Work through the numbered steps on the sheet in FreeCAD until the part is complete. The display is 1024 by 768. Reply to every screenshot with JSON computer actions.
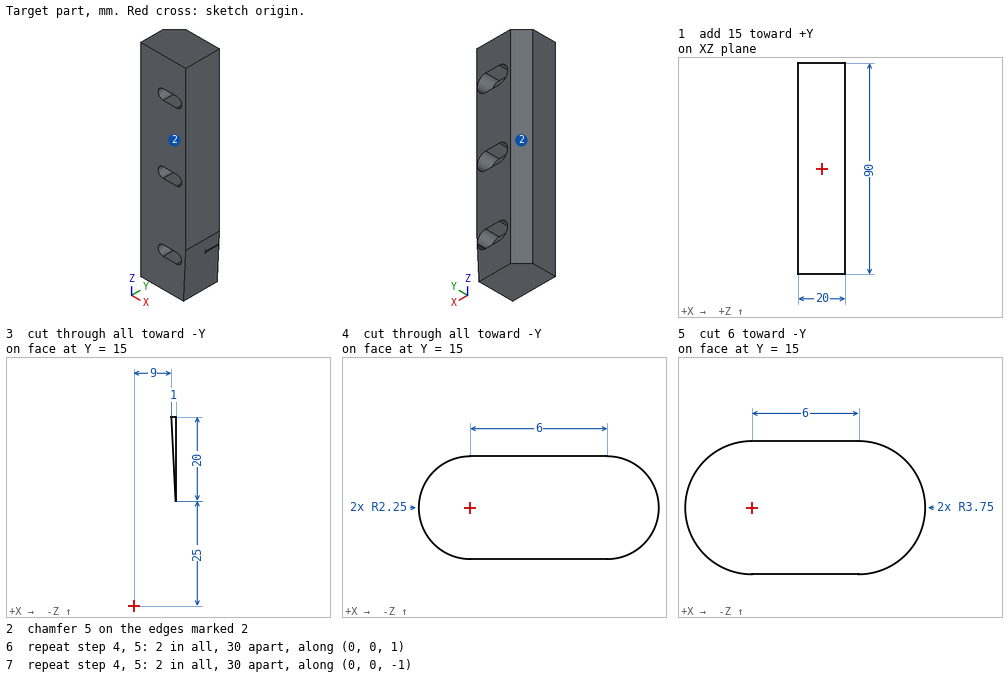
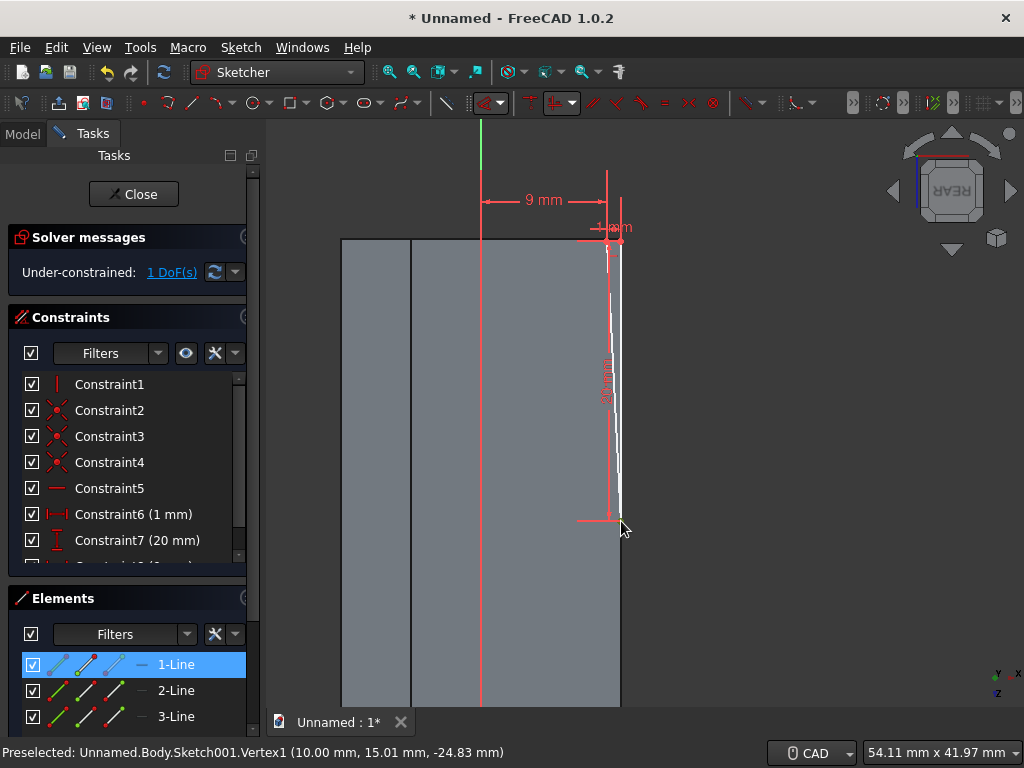
{"action": "key", "text": "i"}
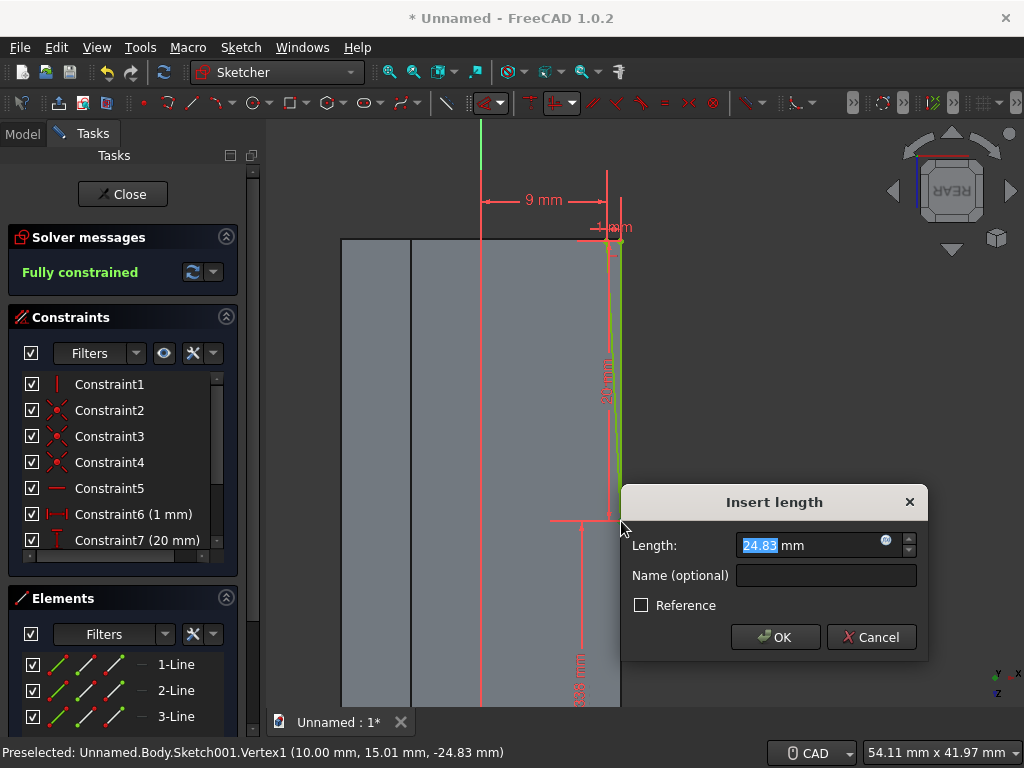
{"action": "type", "text": "25"}
{"action": "key", "text": "Return"}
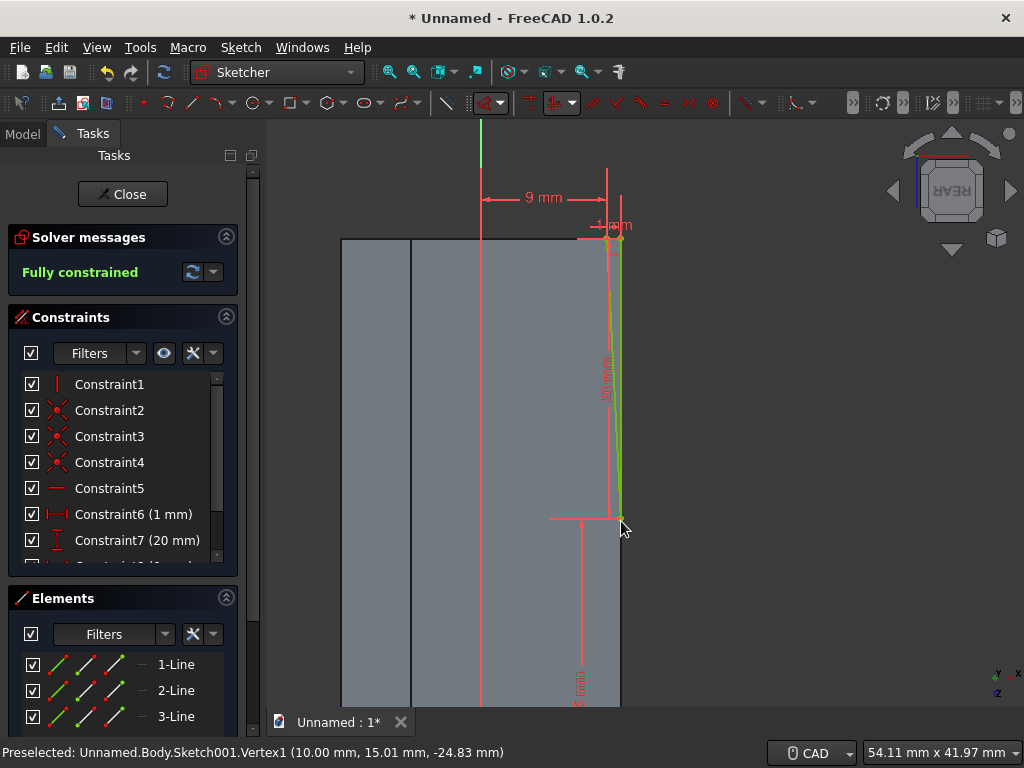
{"action": "left_click", "coordinate": [123, 194]}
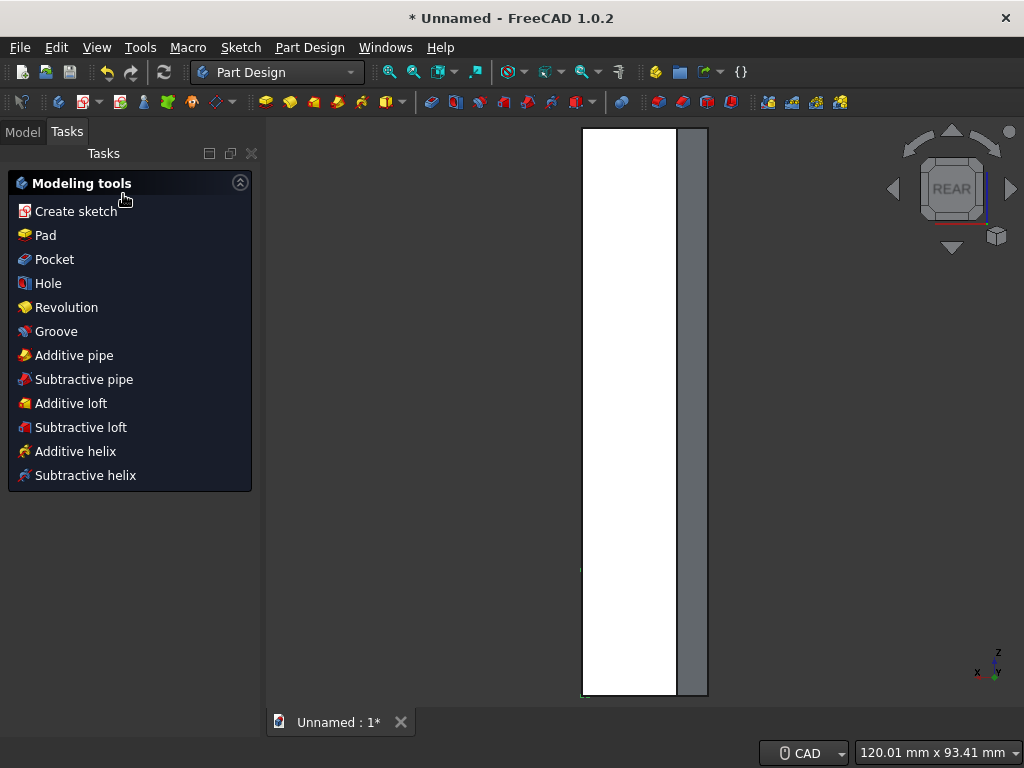
{"action": "left_click", "coordinate": [432, 102]}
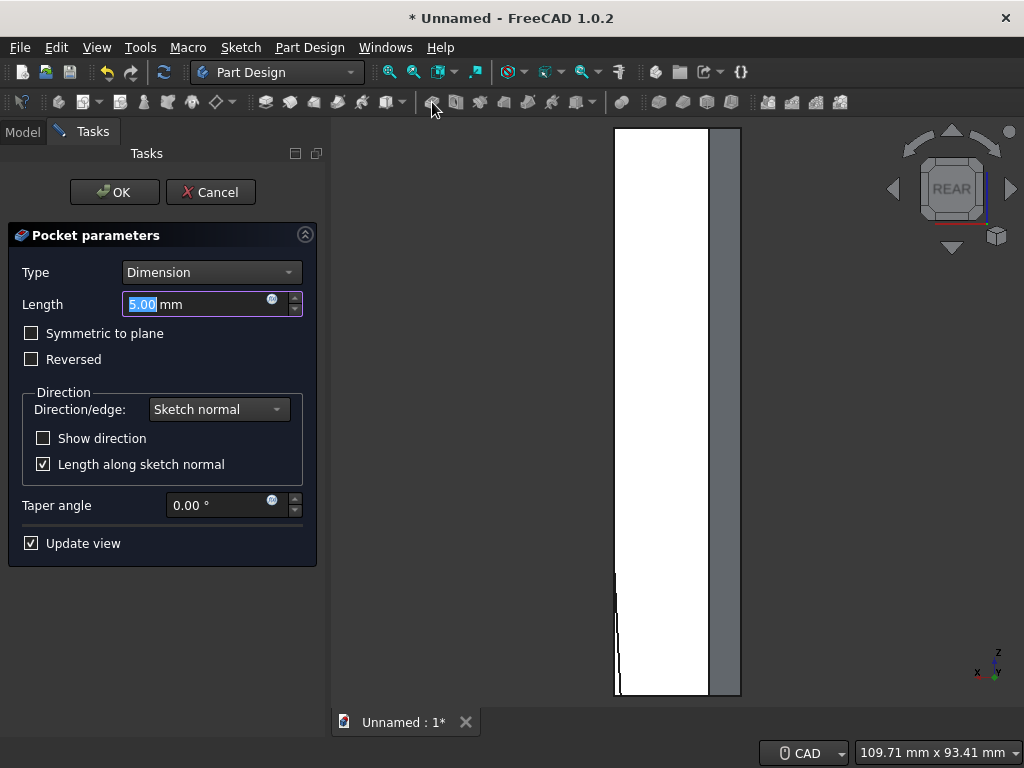
{"action": "left_click", "coordinate": [212, 272]}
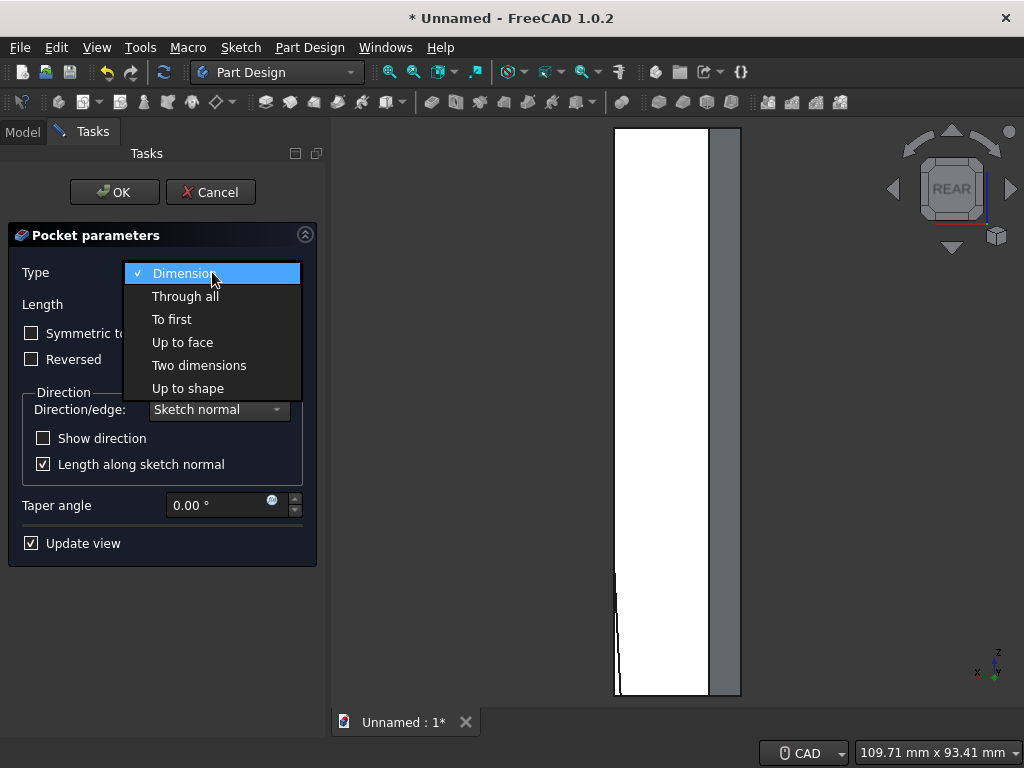
{"action": "left_click", "coordinate": [212, 296]}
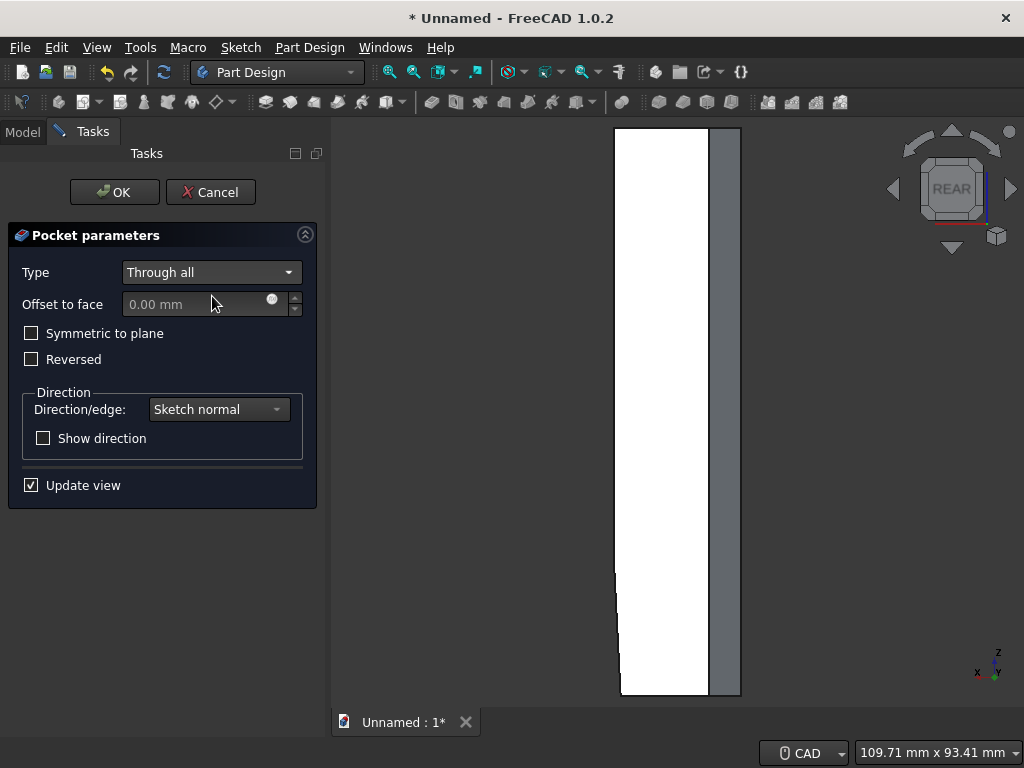
{"action": "left_click", "coordinate": [115, 192]}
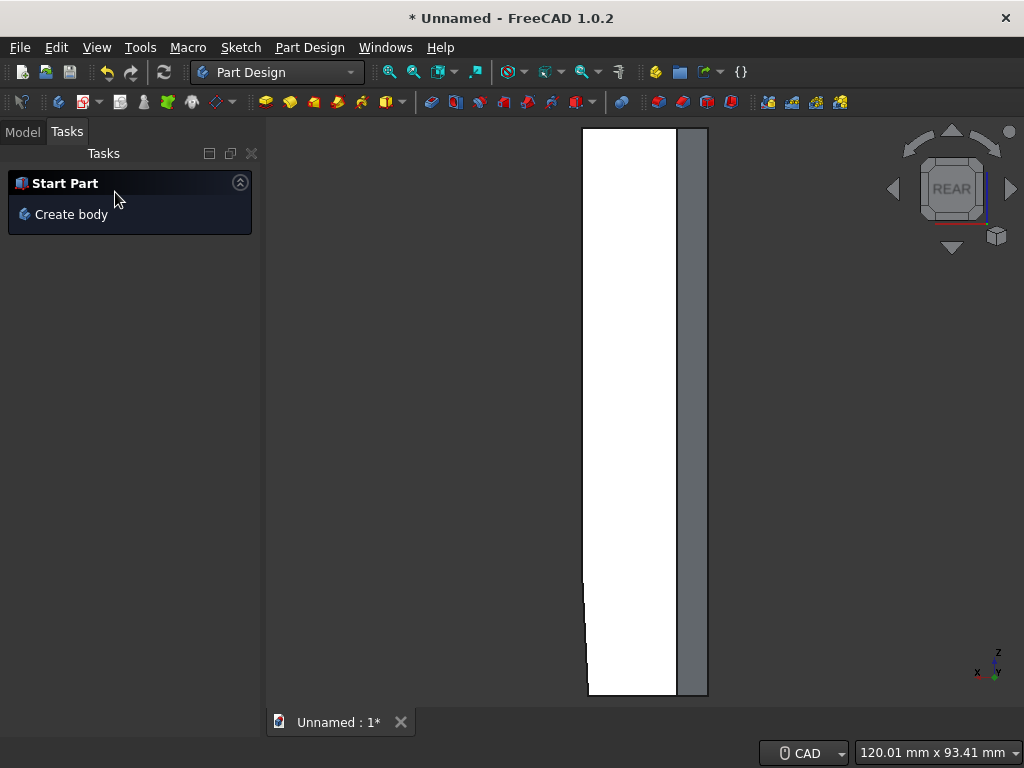
{"action": "left_click", "coordinate": [629, 249]}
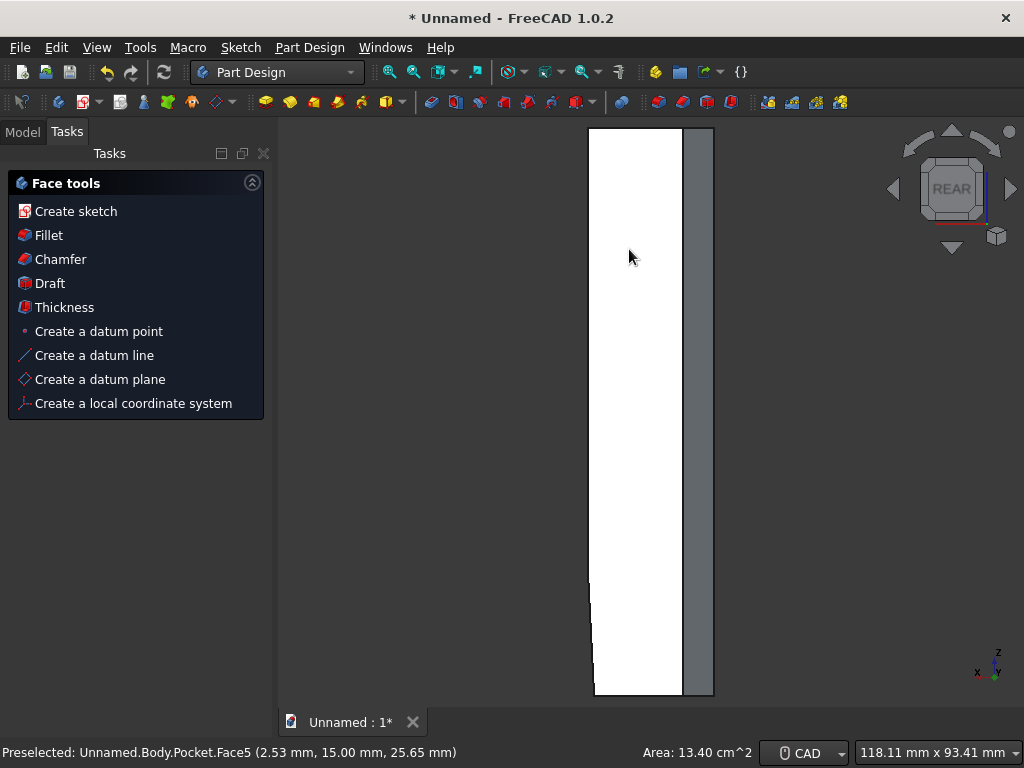
{"action": "left_click", "coordinate": [84, 102]}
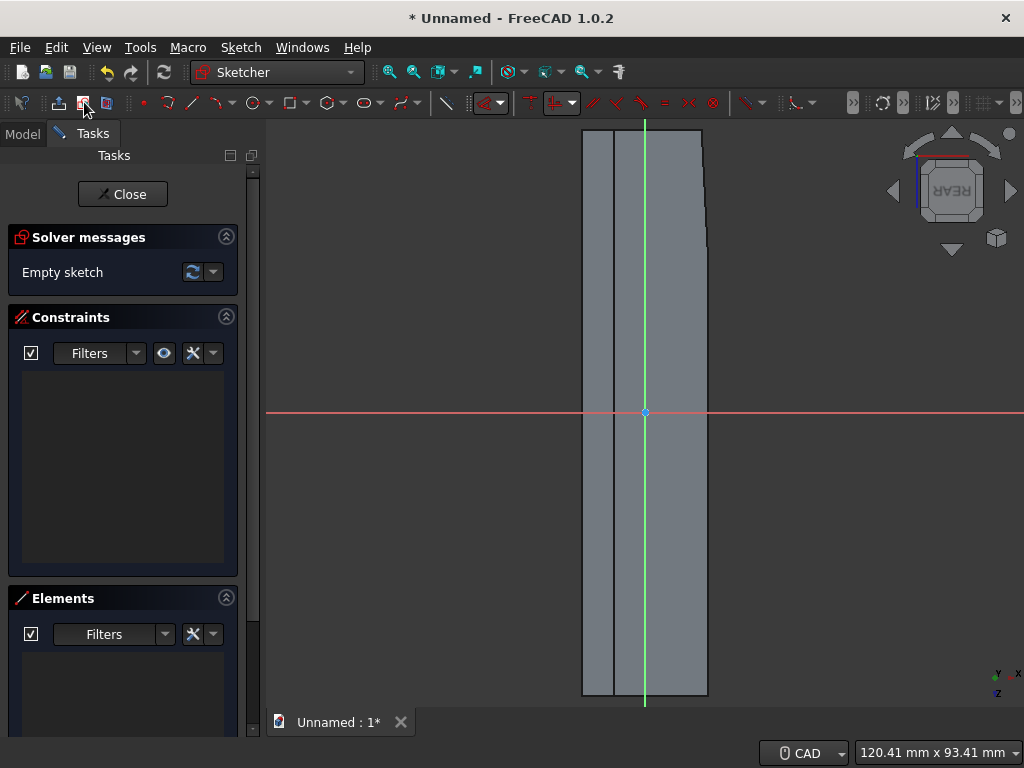
{"action": "scroll", "coordinate": [681, 413], "scroll_direction": "up", "scroll_amount": 9}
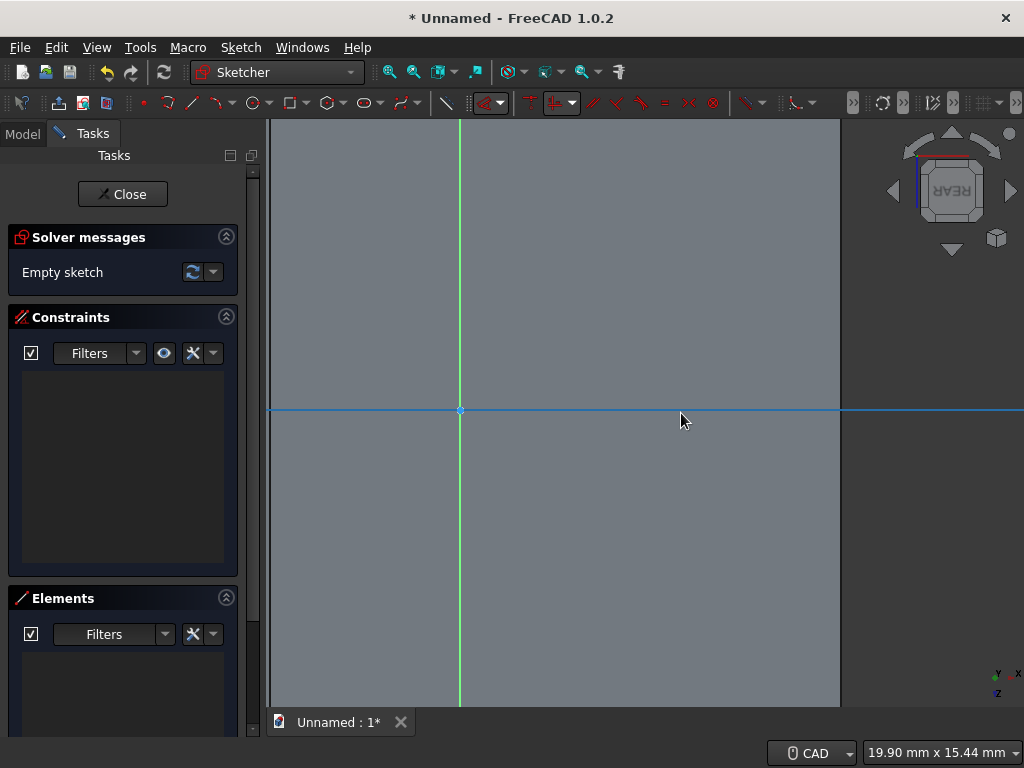
{"action": "left_click", "coordinate": [364, 104]}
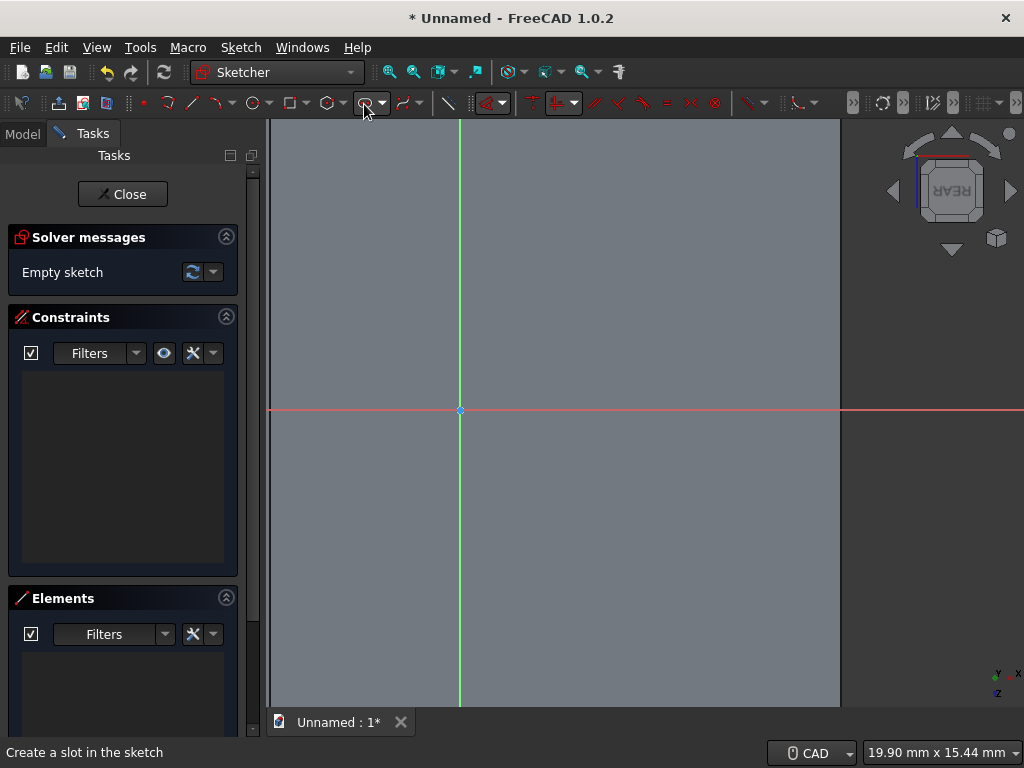
{"action": "left_click", "coordinate": [460, 410]}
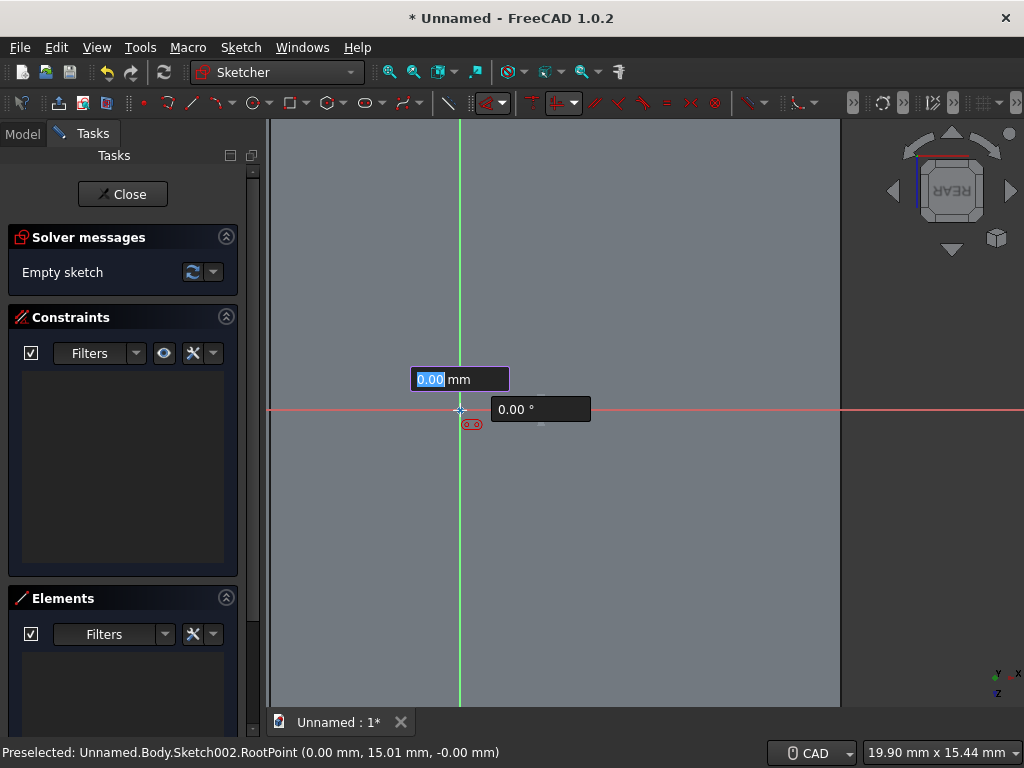
{"action": "left_click", "coordinate": [689, 401]}